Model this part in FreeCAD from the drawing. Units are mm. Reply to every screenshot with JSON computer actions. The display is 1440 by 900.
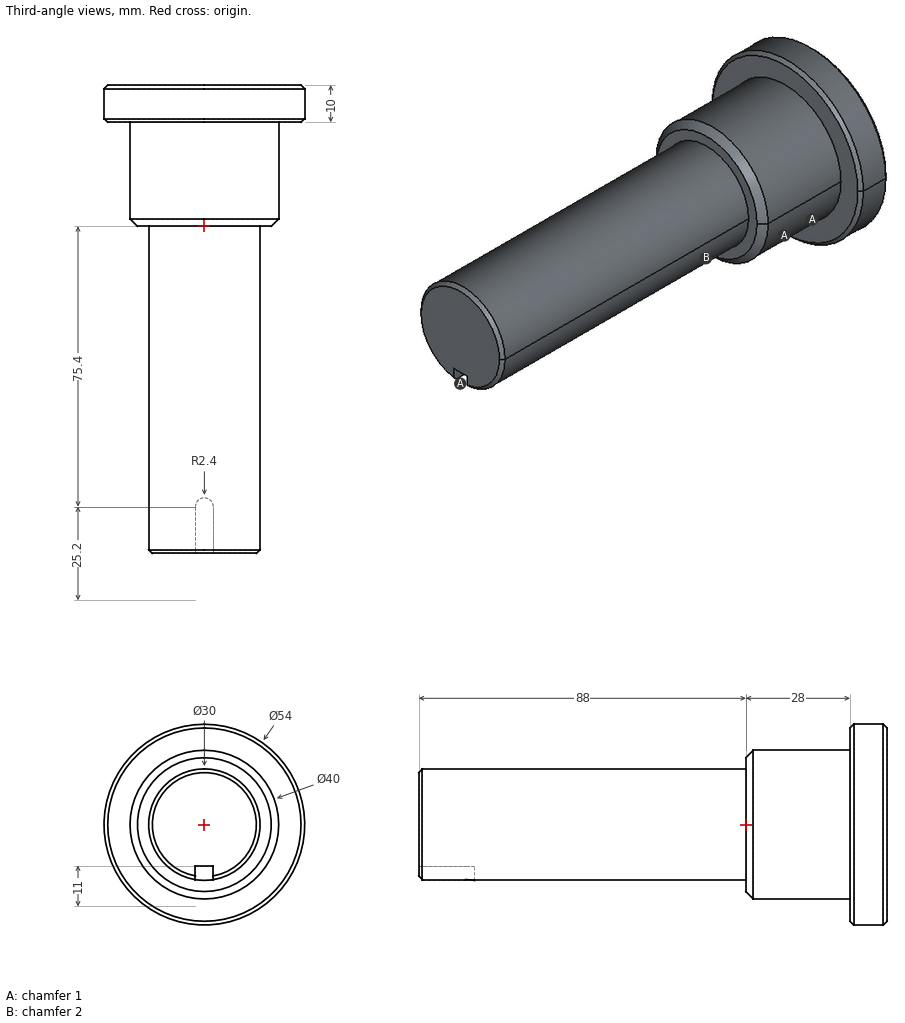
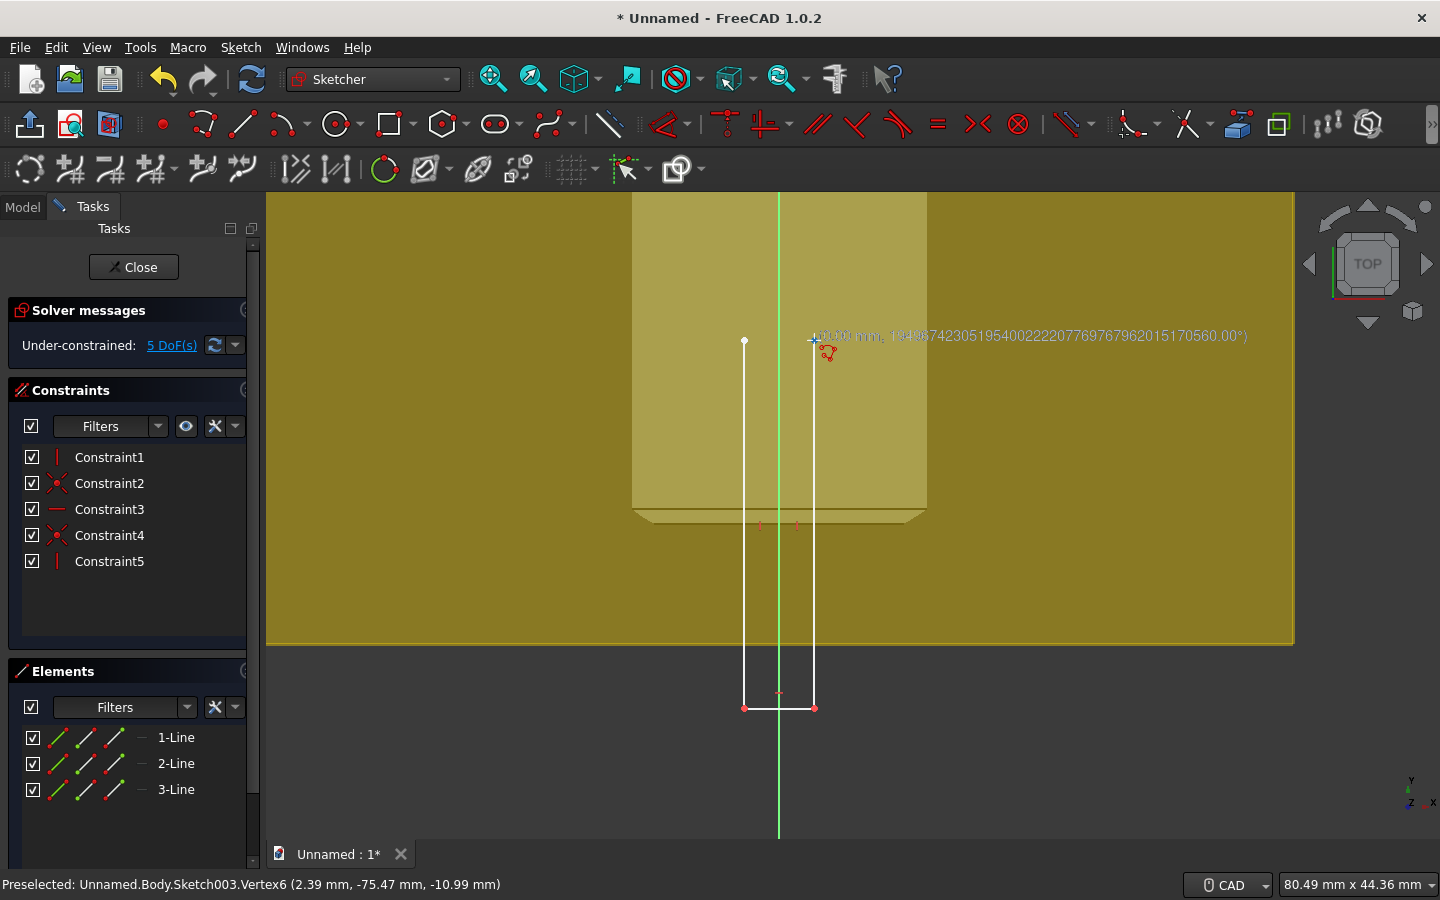
{"action": "key", "text": "g 3 a"}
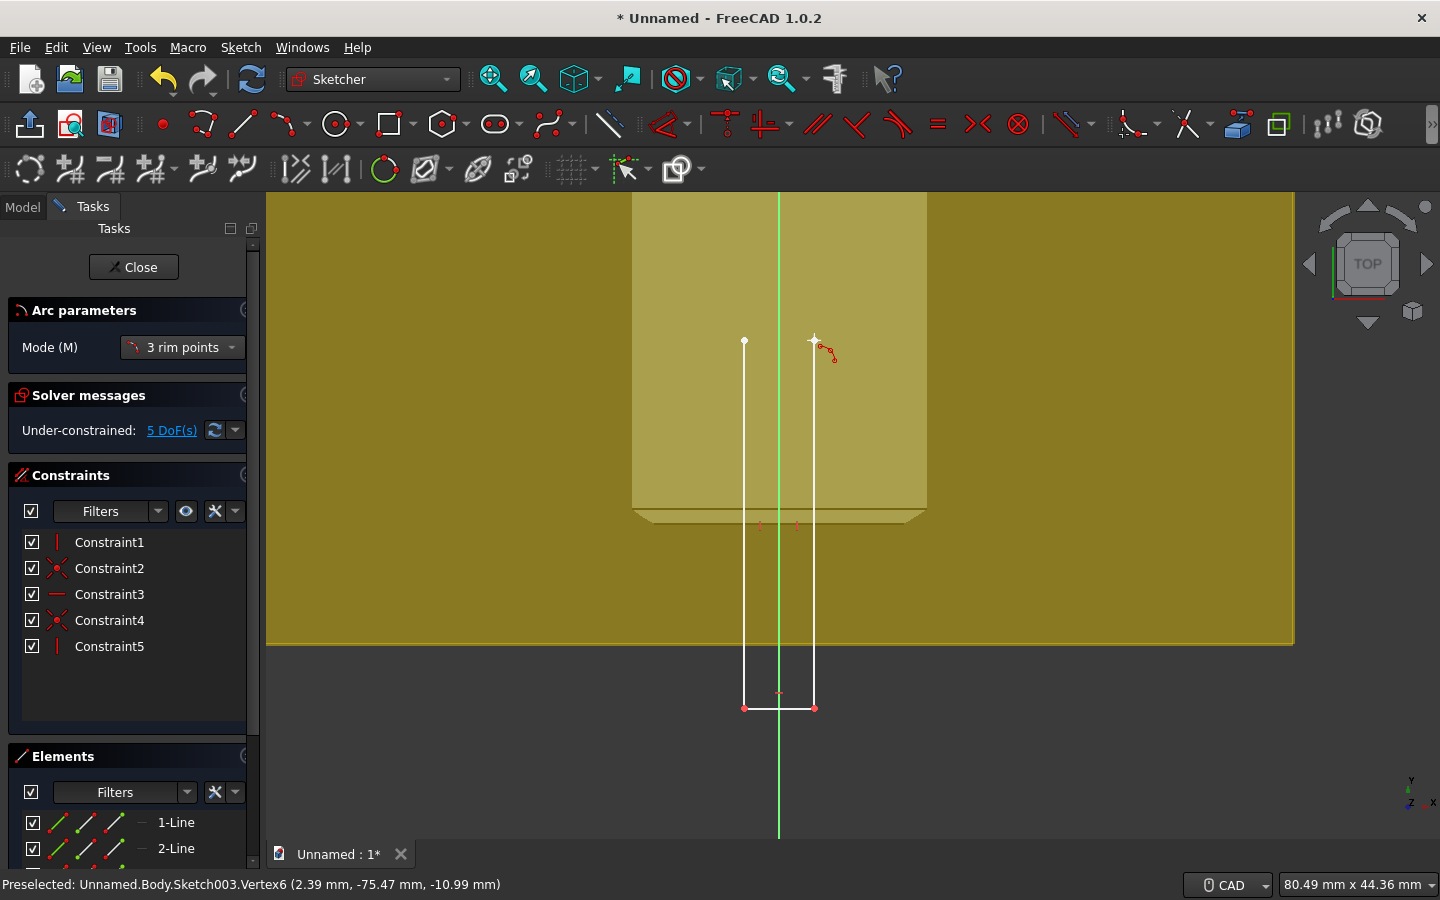
{"action": "left_click", "coordinate": [814, 341]}
{"action": "left_click", "coordinate": [744, 341]}
{"action": "left_click", "coordinate": [800, 312]}
{"action": "key", "text": "Escape"}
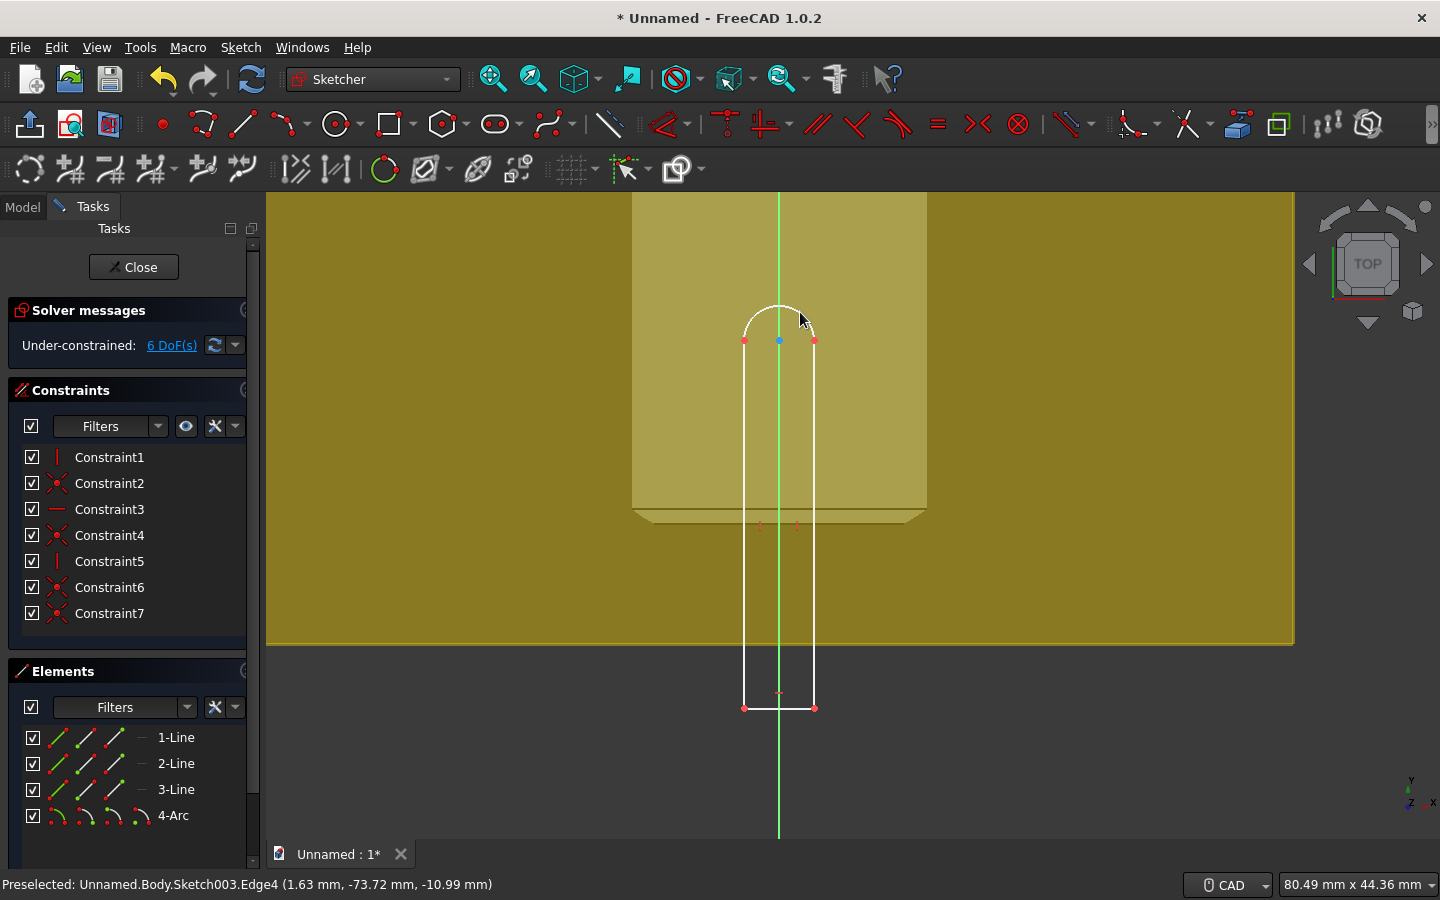
{"action": "left_click", "coordinate": [744, 451]}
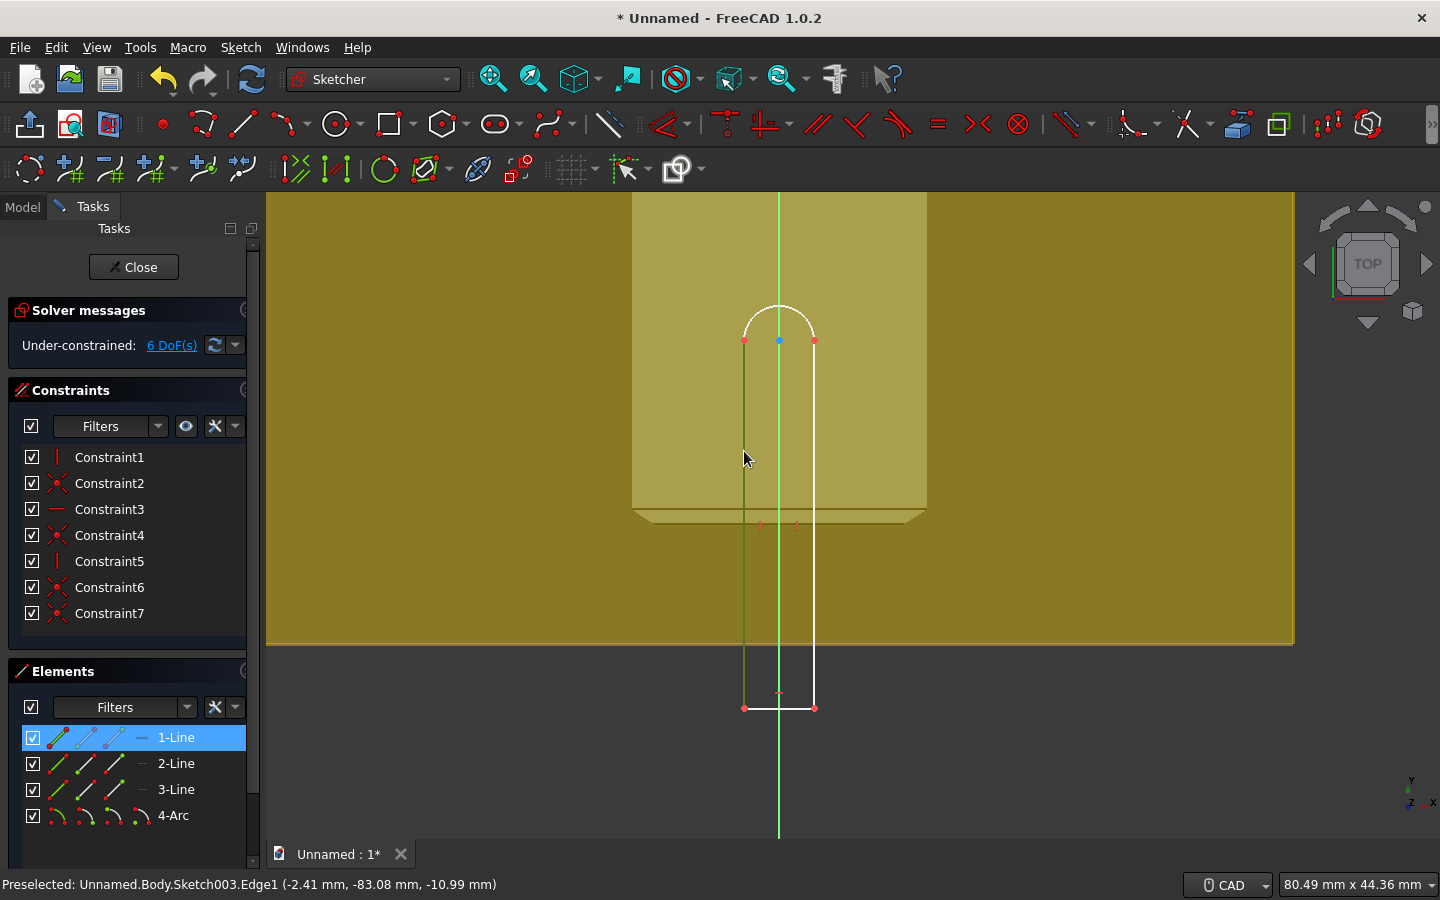
{"action": "left_click", "coordinate": [800, 313]}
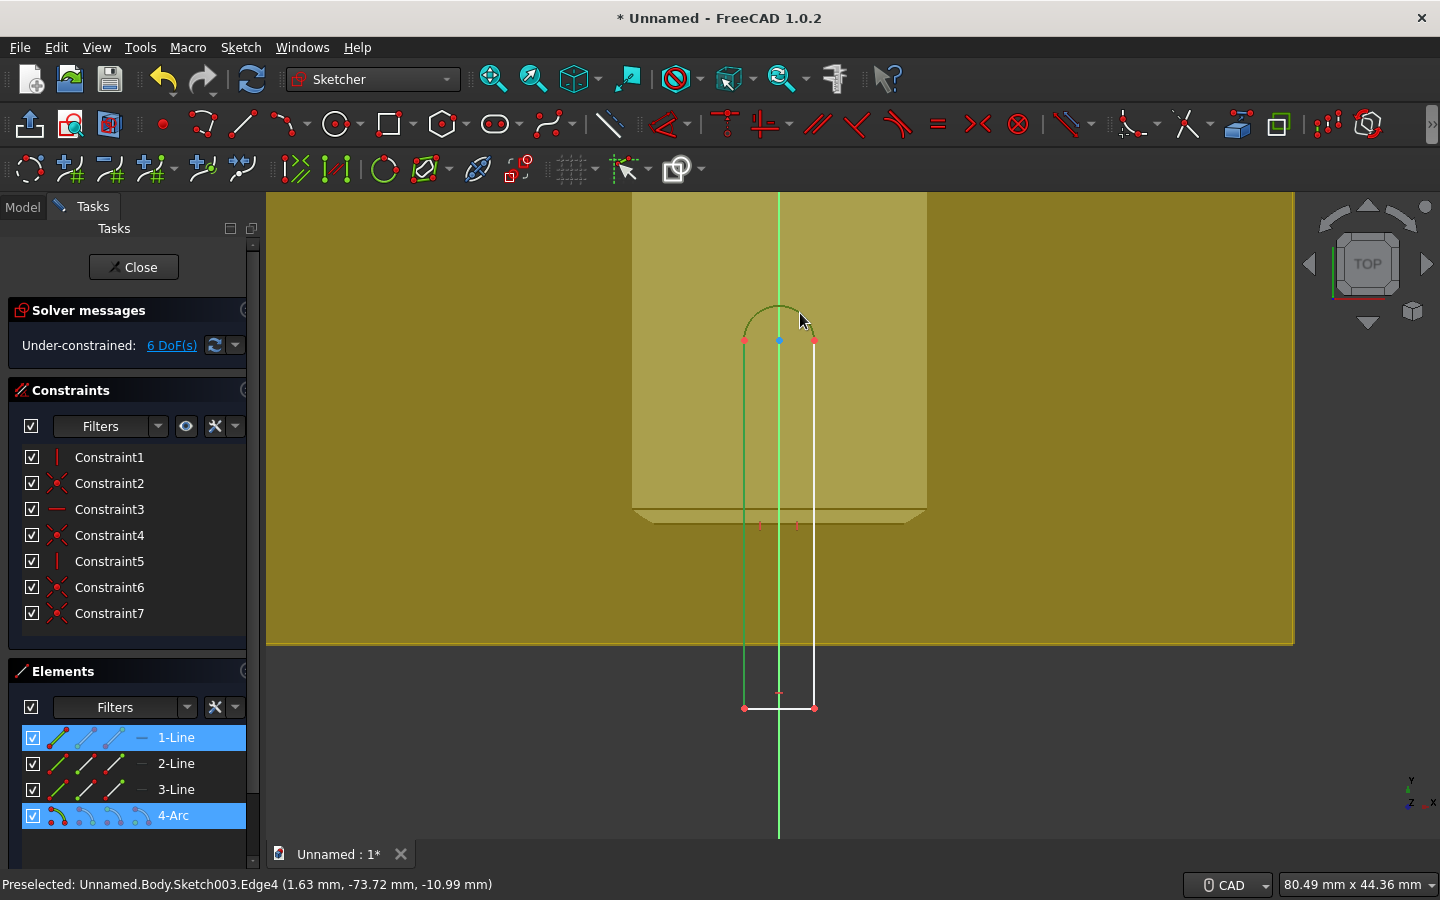
{"action": "key", "text": "t"}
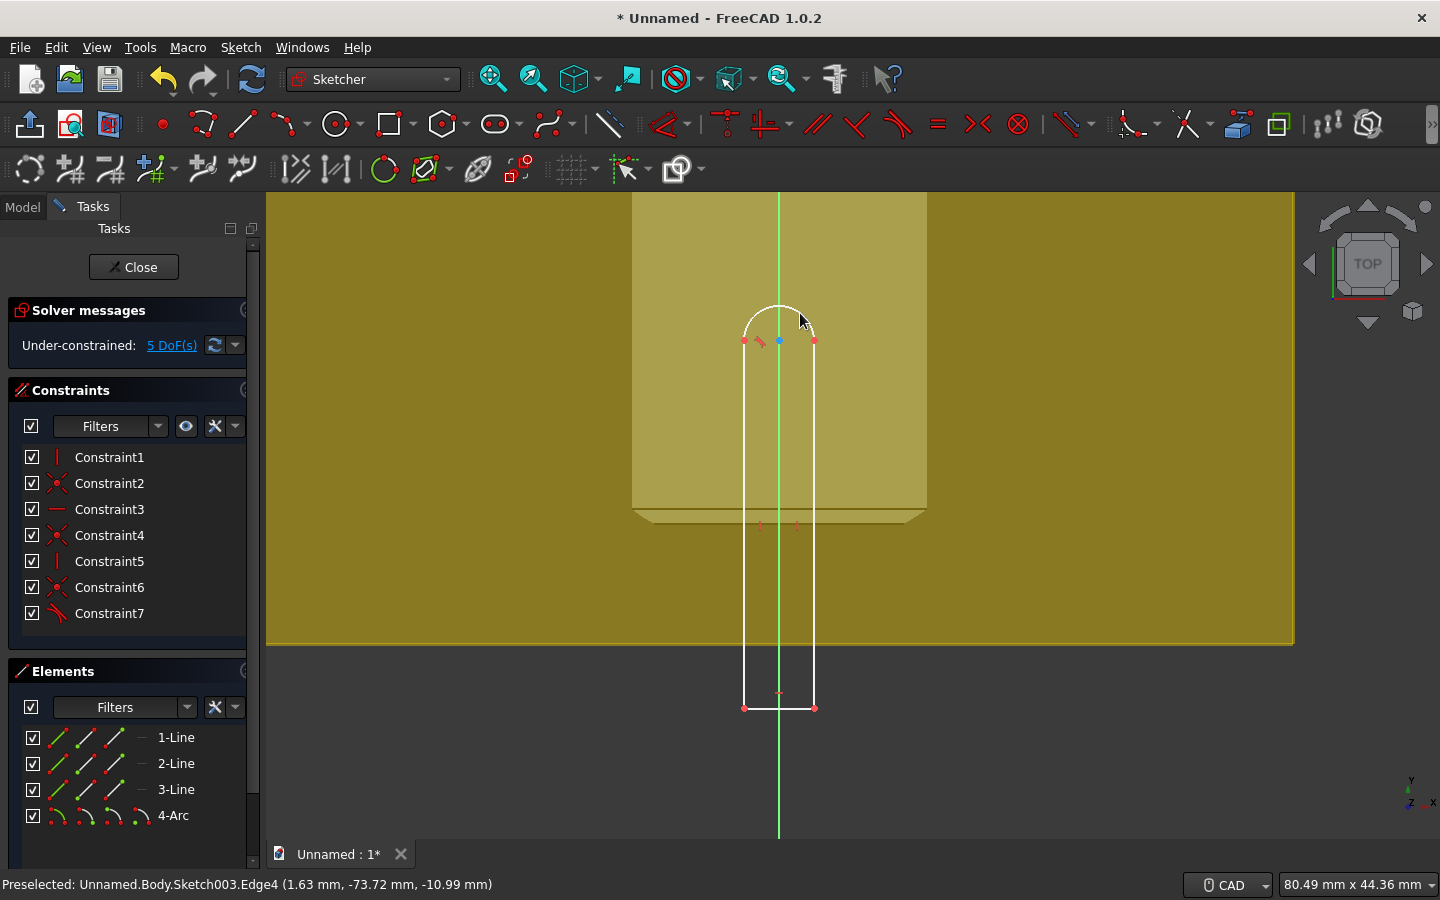
{"action": "left_click", "coordinate": [814, 599]}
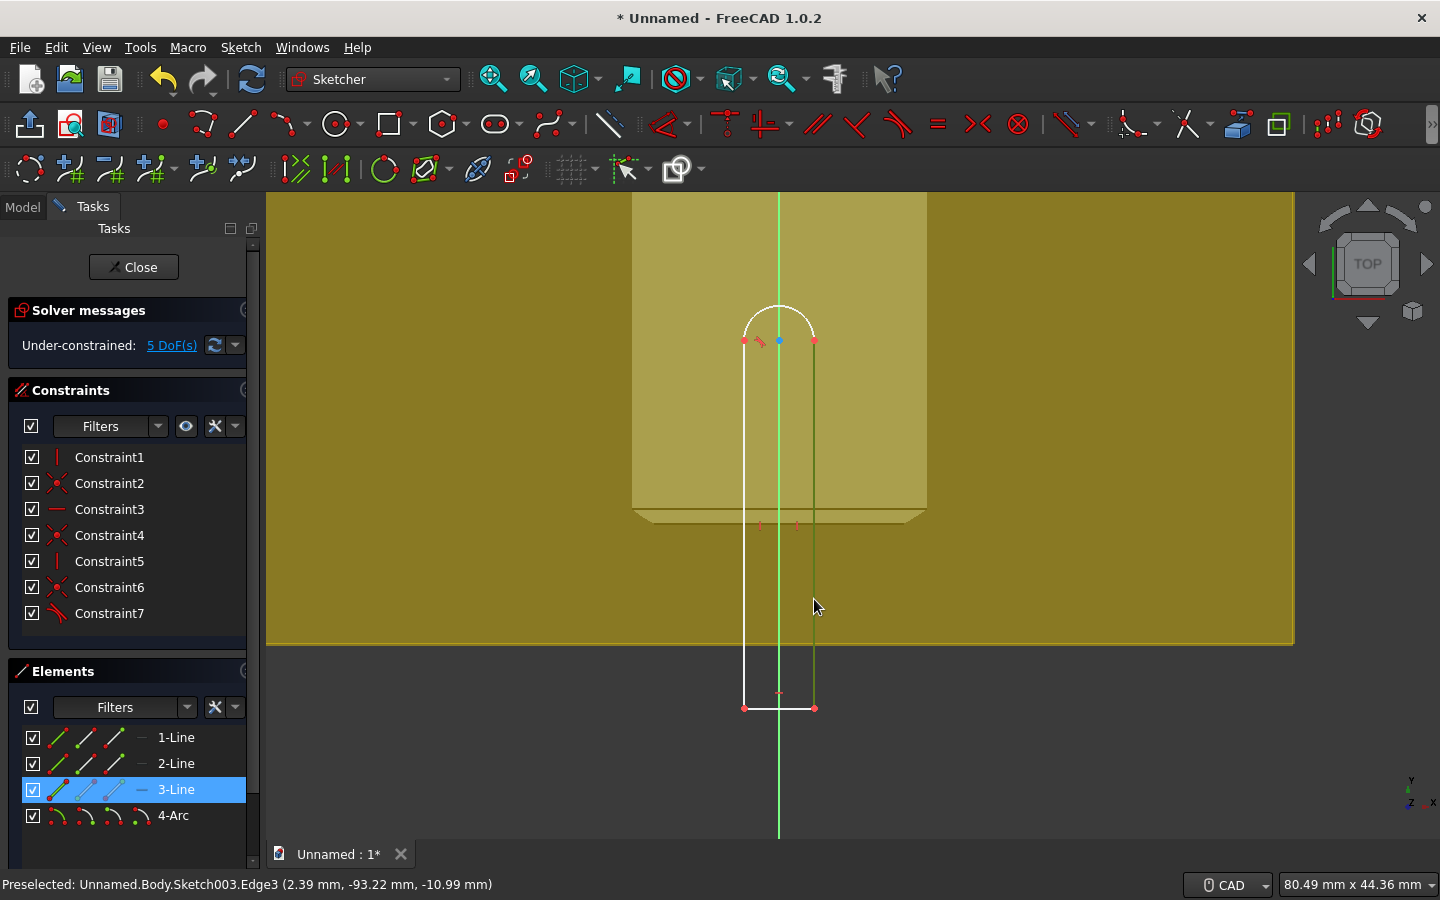
{"action": "left_click", "coordinate": [800, 313]}